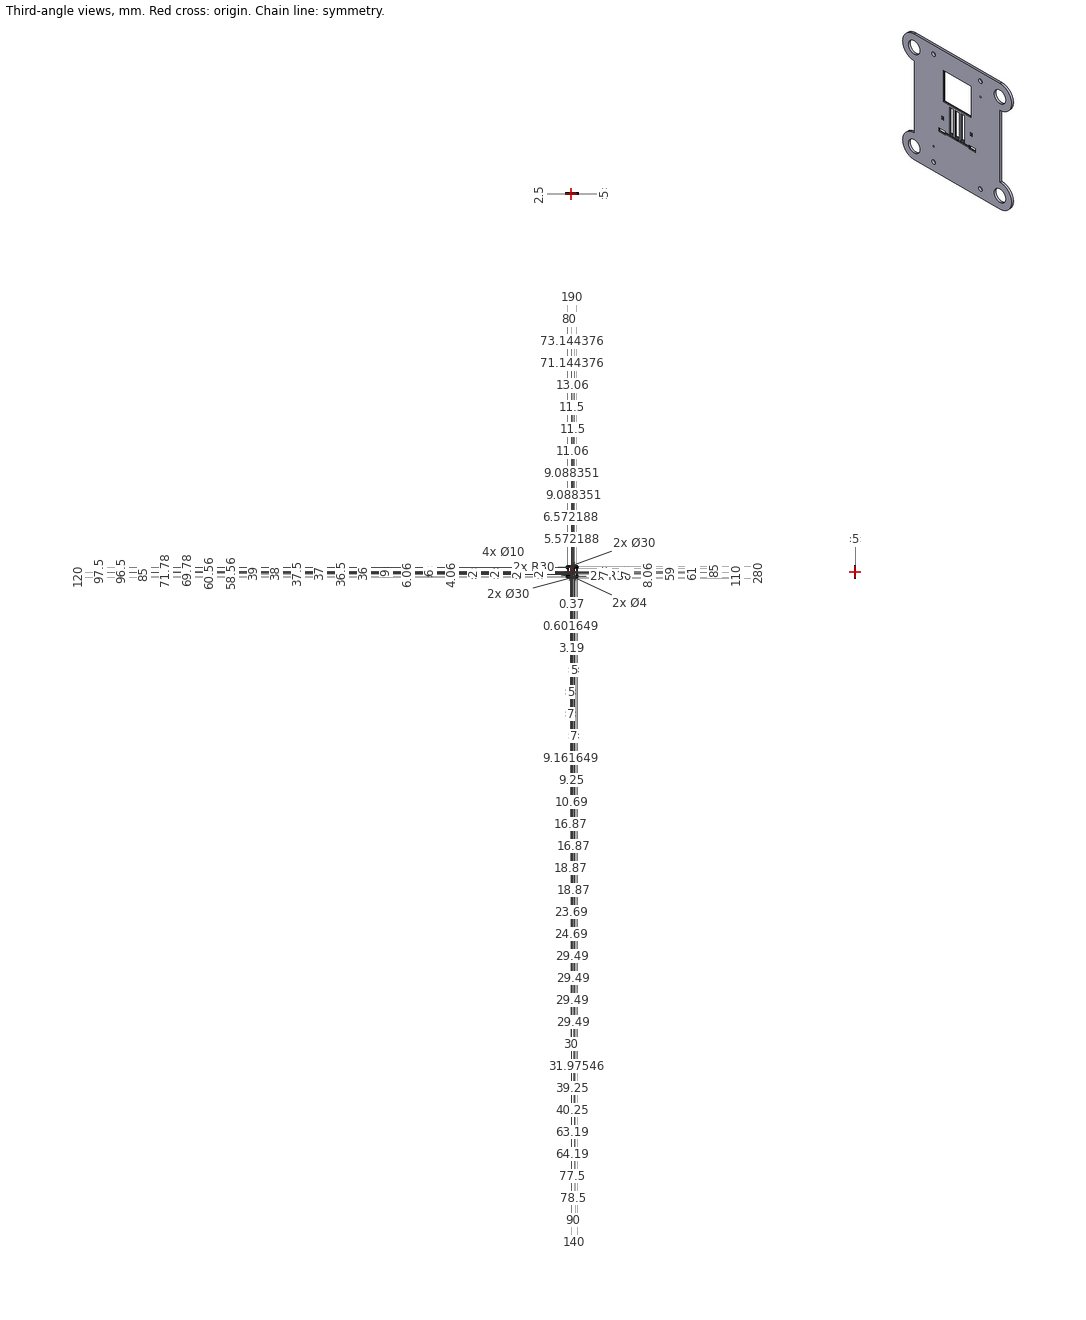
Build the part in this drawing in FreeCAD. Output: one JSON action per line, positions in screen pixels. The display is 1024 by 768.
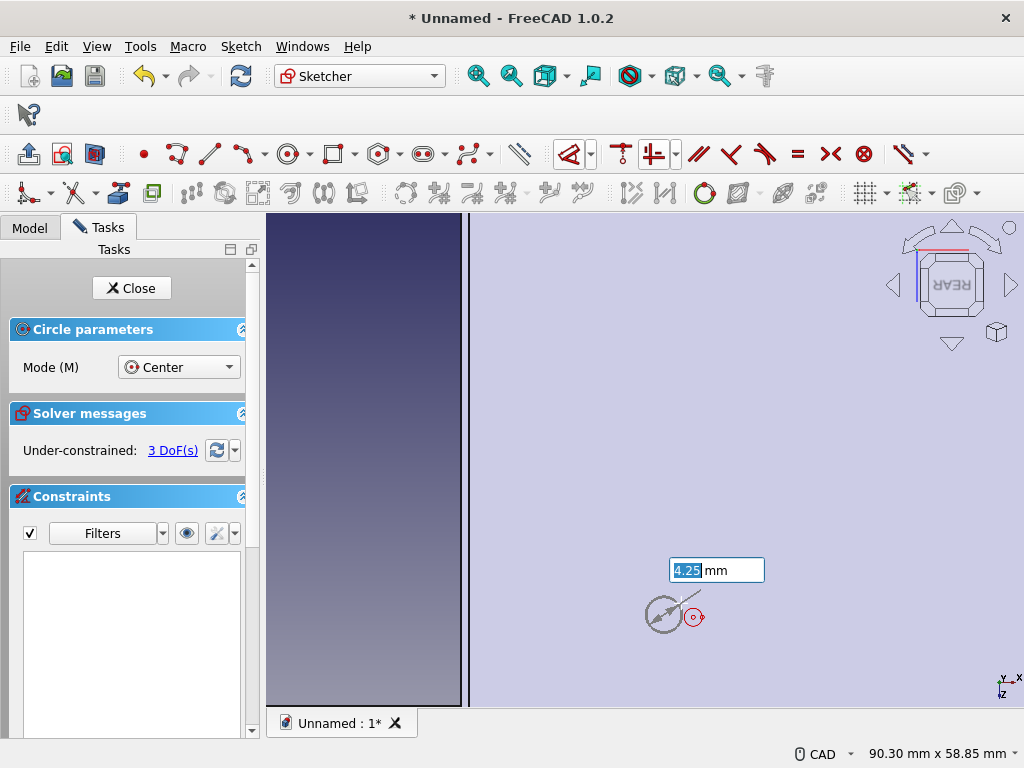
{"action": "left_click", "coordinate": [678, 598]}
{"action": "key", "text": "Escape"}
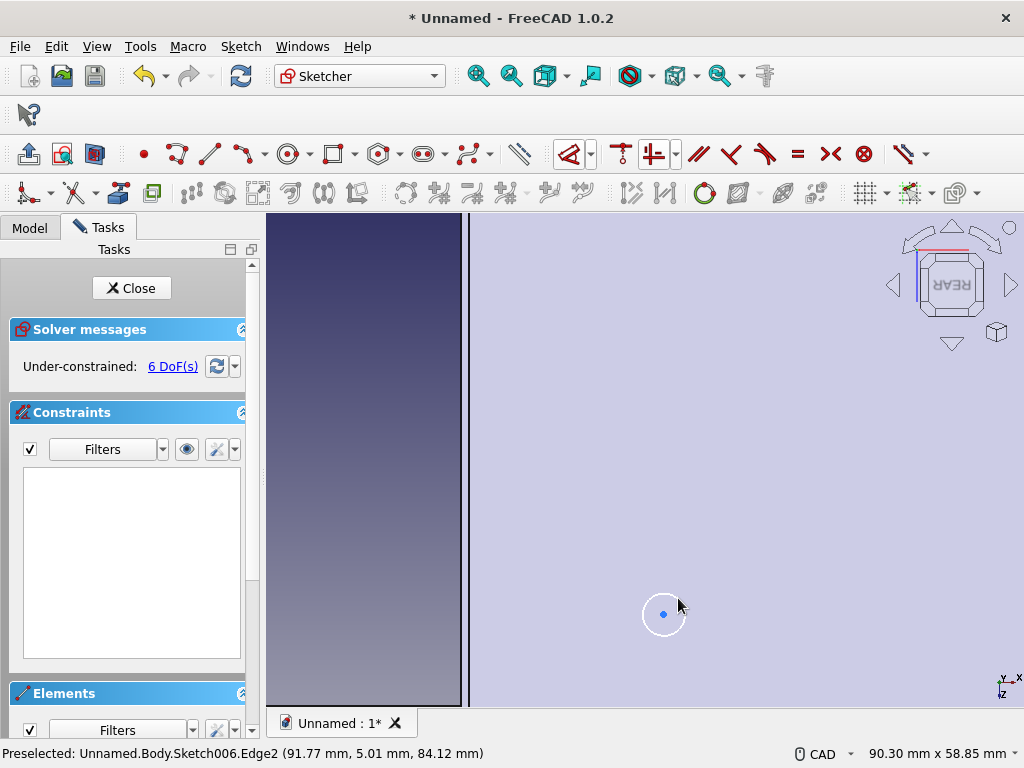
{"action": "scroll", "coordinate": [681, 603], "scroll_direction": "down", "scroll_amount": 8}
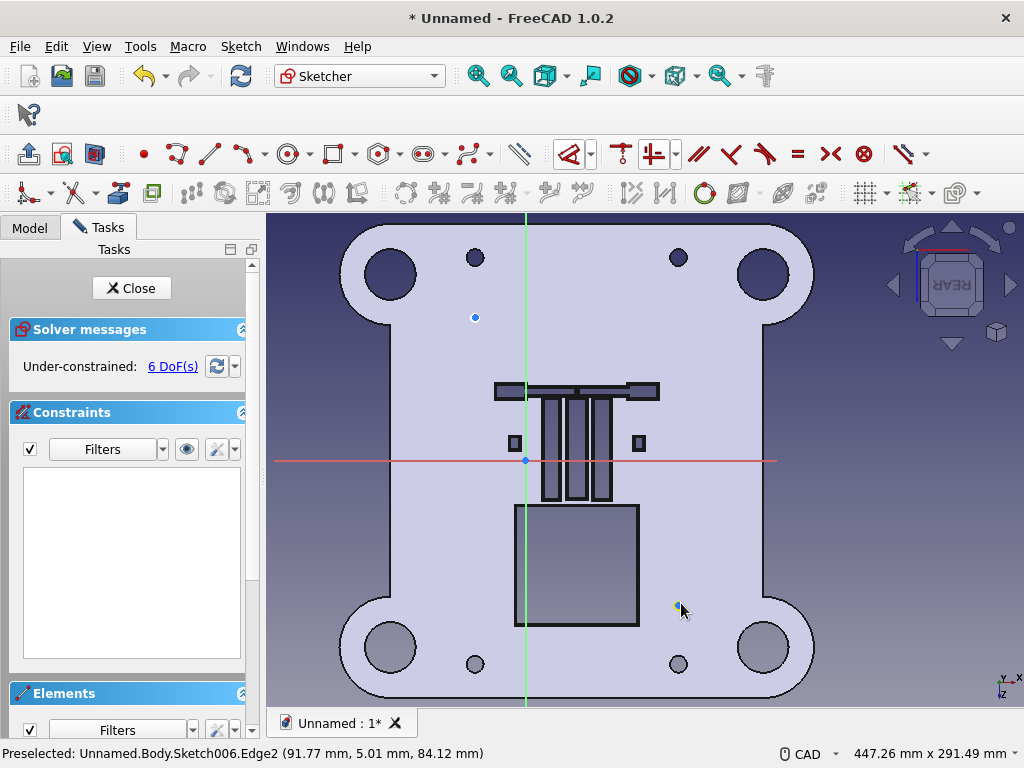
{"action": "scroll", "coordinate": [478, 315], "scroll_direction": "up", "scroll_amount": 7}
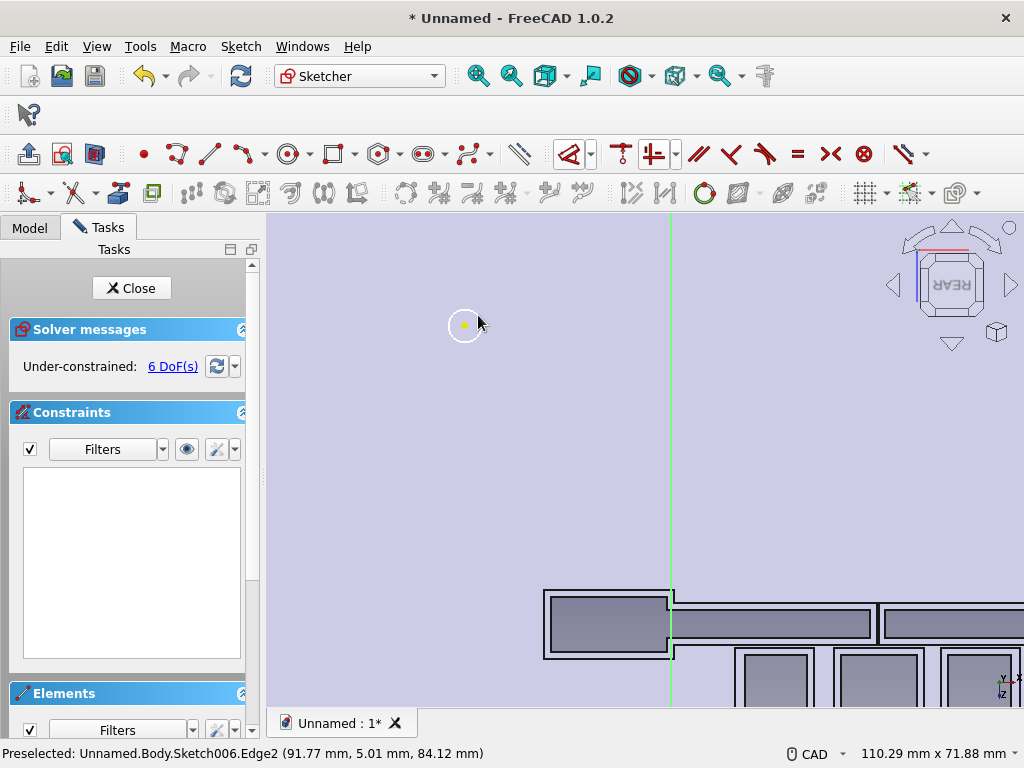
{"action": "left_click", "coordinate": [477, 314]}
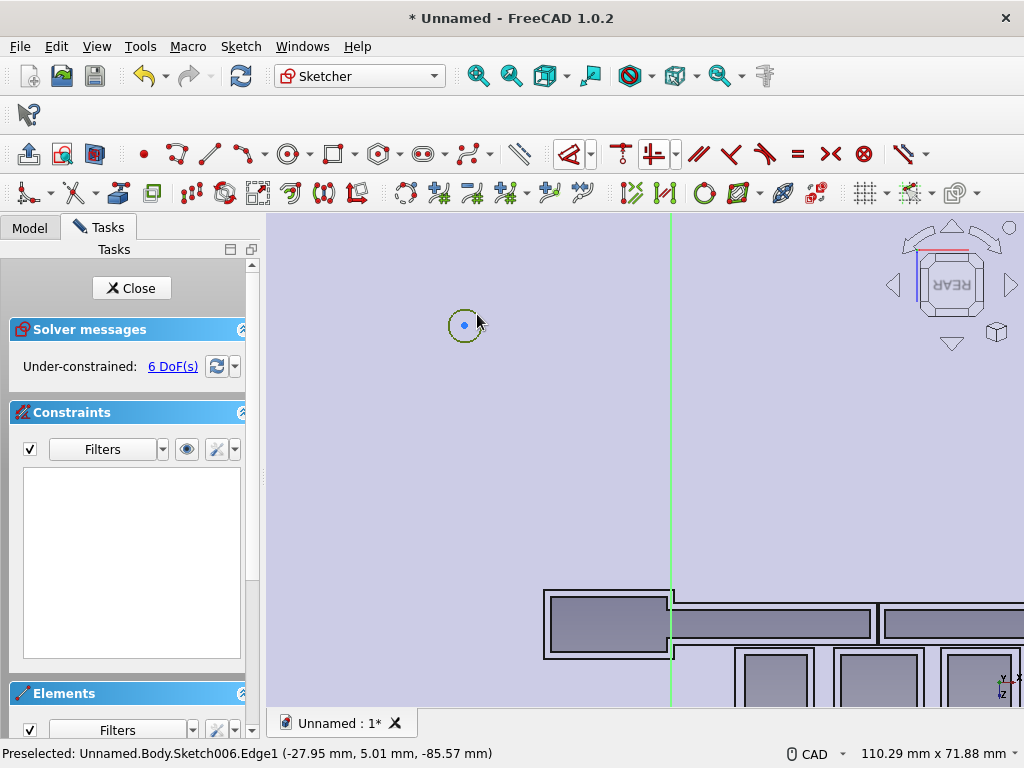
{"action": "scroll", "coordinate": [478, 314], "scroll_direction": "down", "scroll_amount": 7}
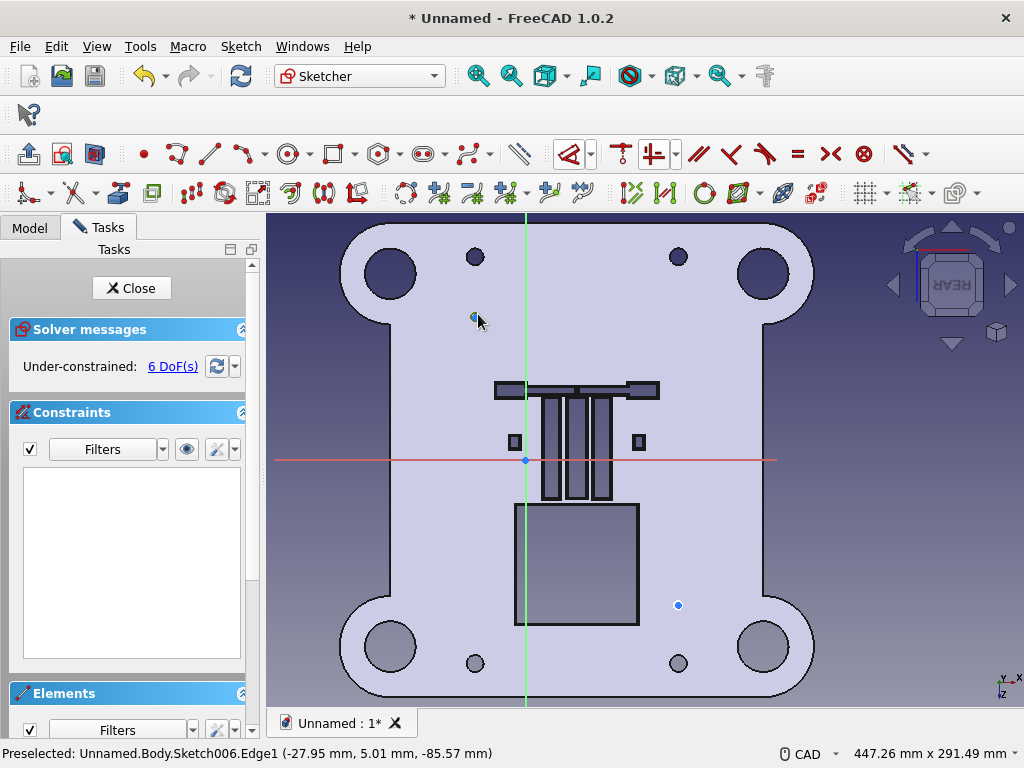
{"action": "scroll", "coordinate": [681, 602], "scroll_direction": "up", "scroll_amount": 6}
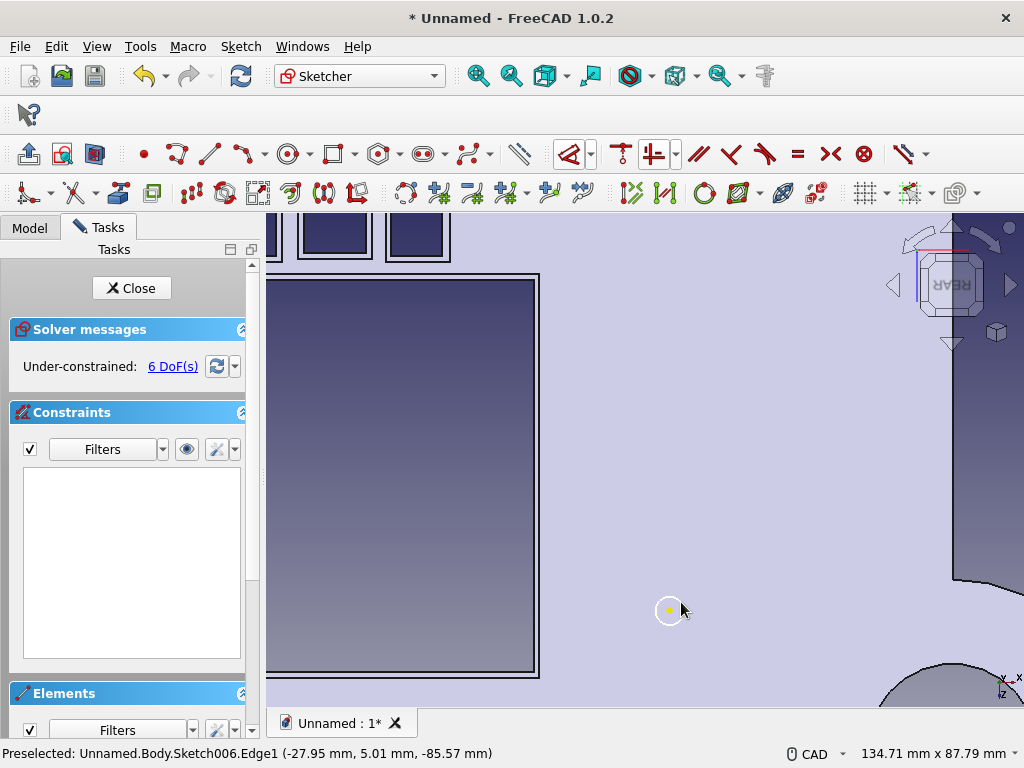
{"action": "left_click", "coordinate": [680, 601]}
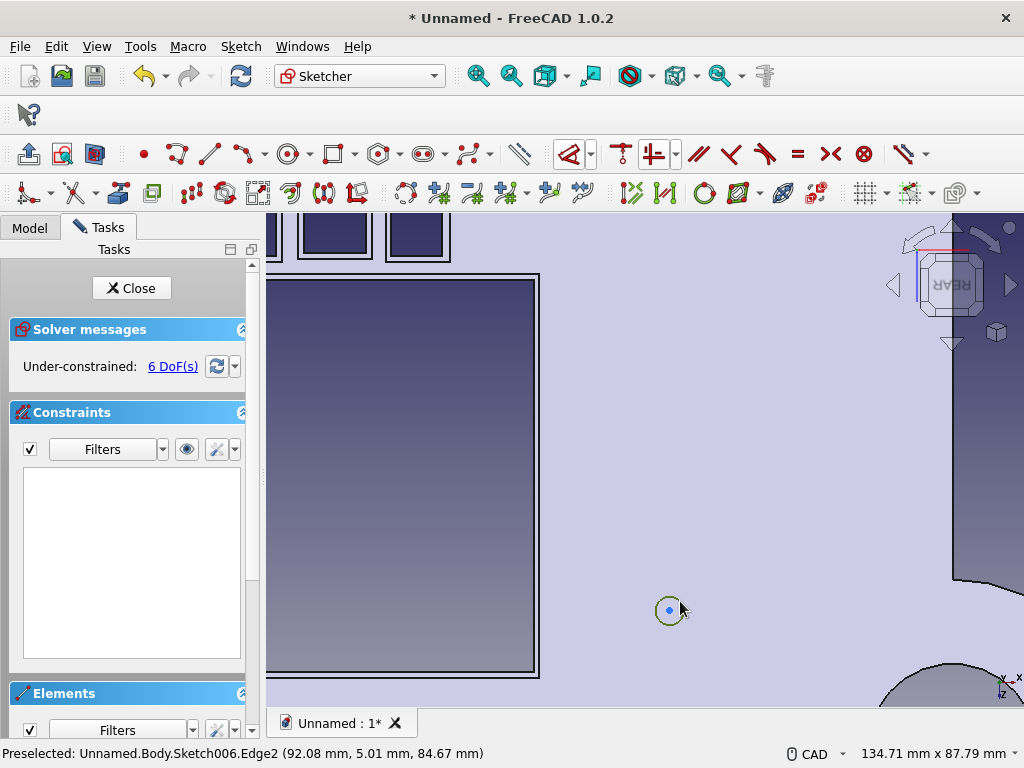
{"action": "key", "text": "e"}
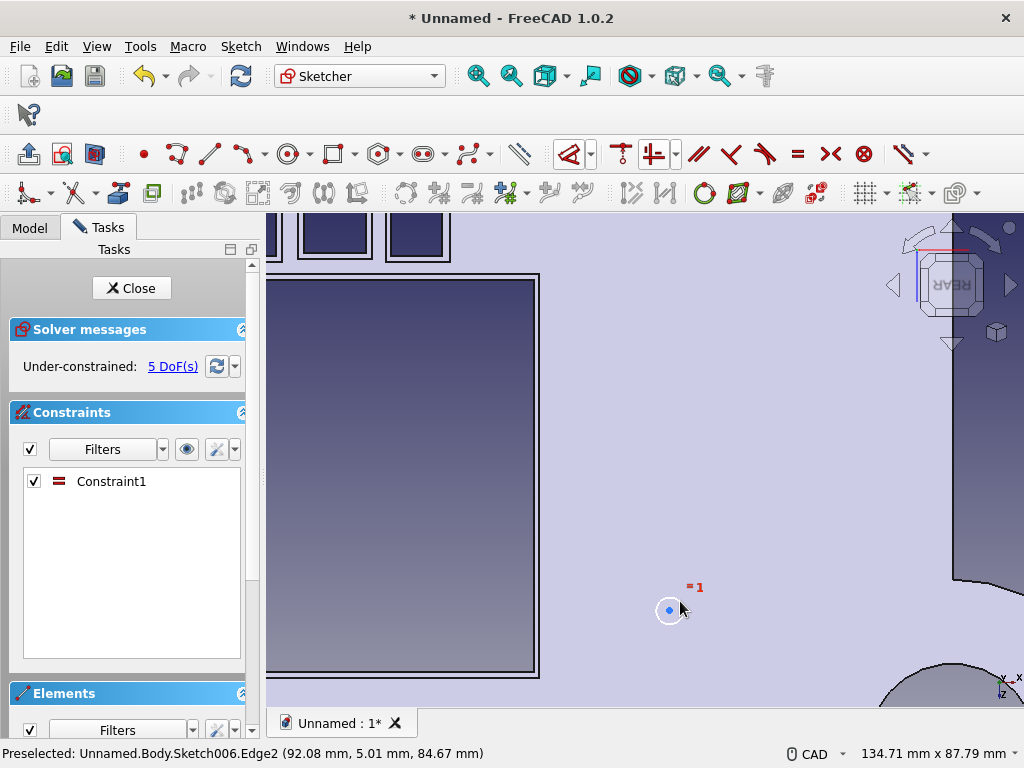
{"action": "scroll", "coordinate": [681, 603], "scroll_direction": "down", "scroll_amount": 6}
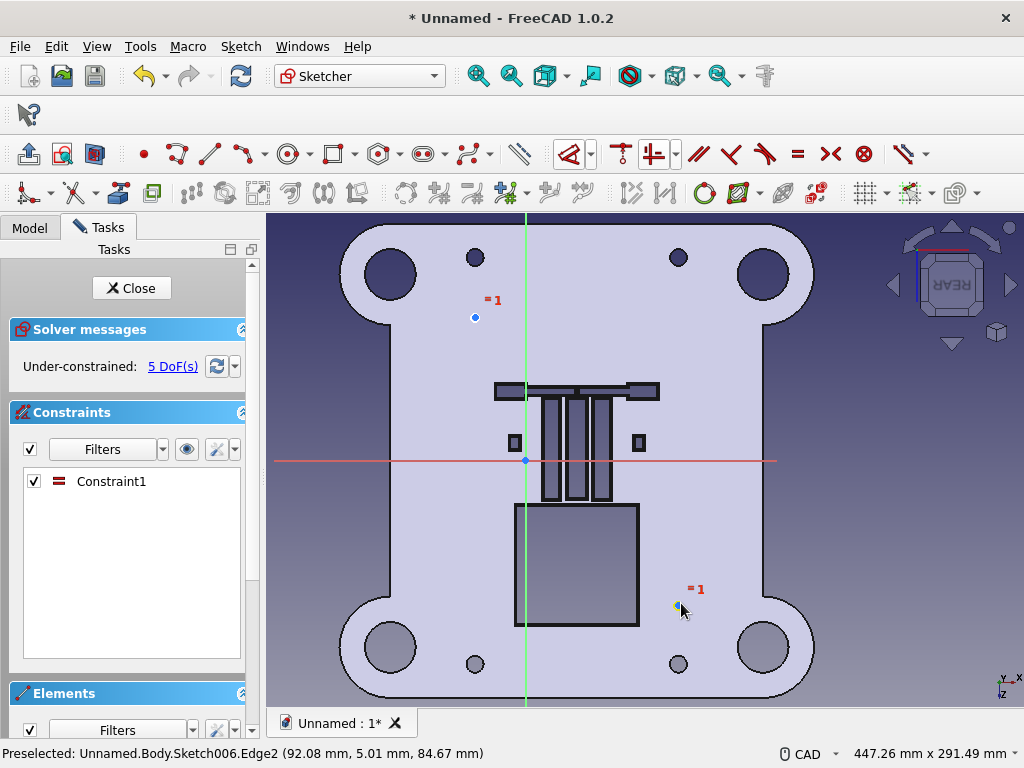
{"action": "scroll", "coordinate": [478, 315], "scroll_direction": "up", "scroll_amount": 9}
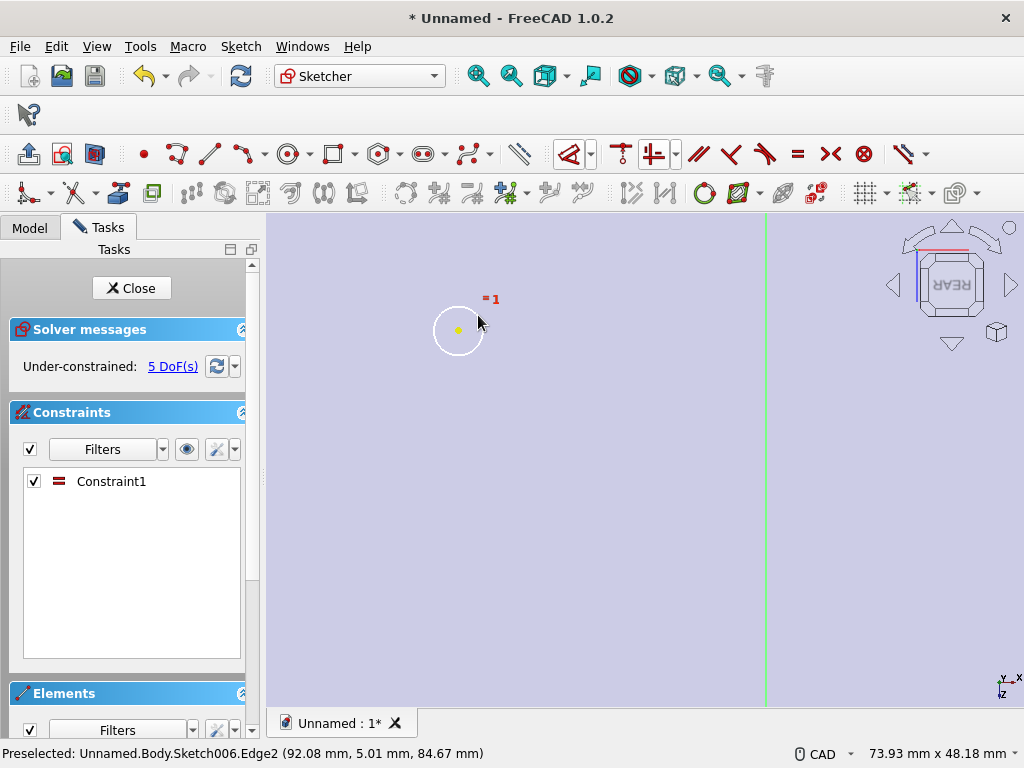
{"action": "left_click", "coordinate": [476, 314]}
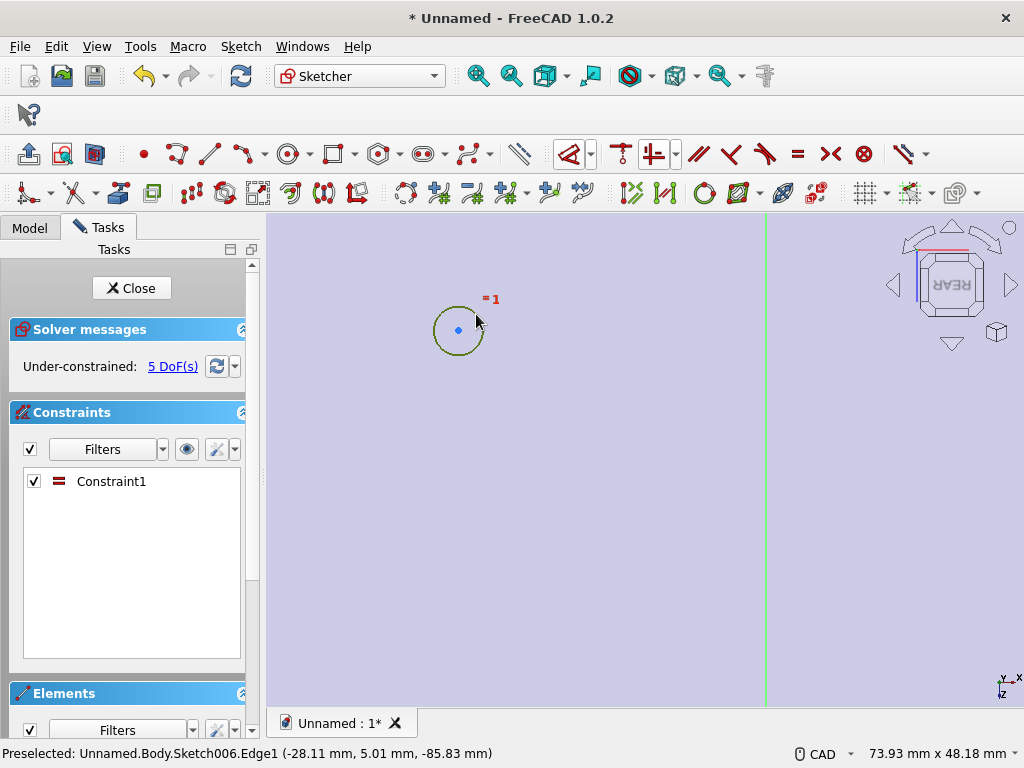
{"action": "left_click", "coordinate": [590, 154]}